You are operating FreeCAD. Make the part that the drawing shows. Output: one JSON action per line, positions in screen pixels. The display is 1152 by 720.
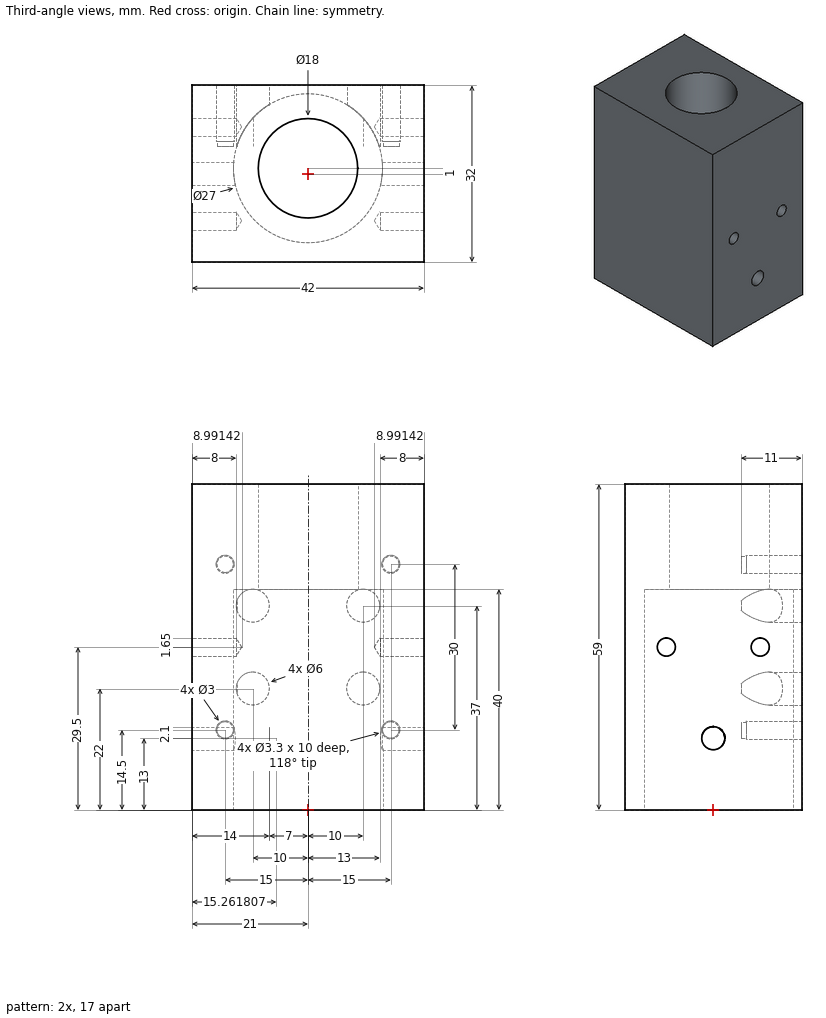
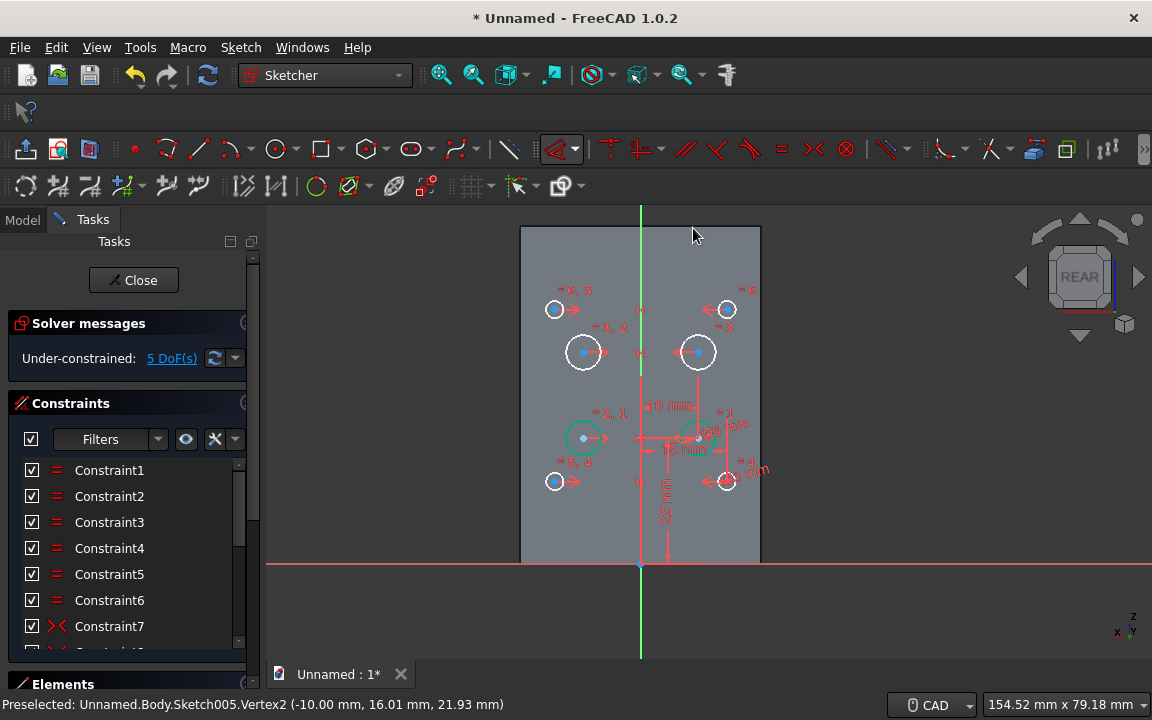
{"action": "left_click", "coordinate": [555, 310]}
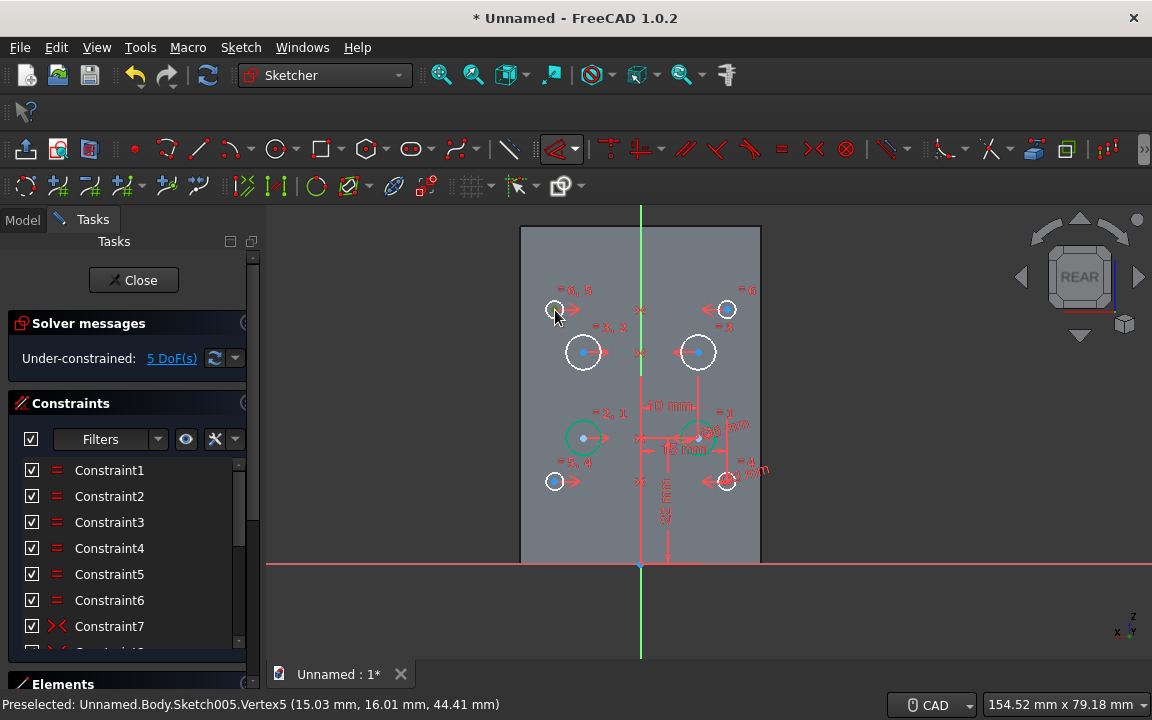
{"action": "key", "text": "l"}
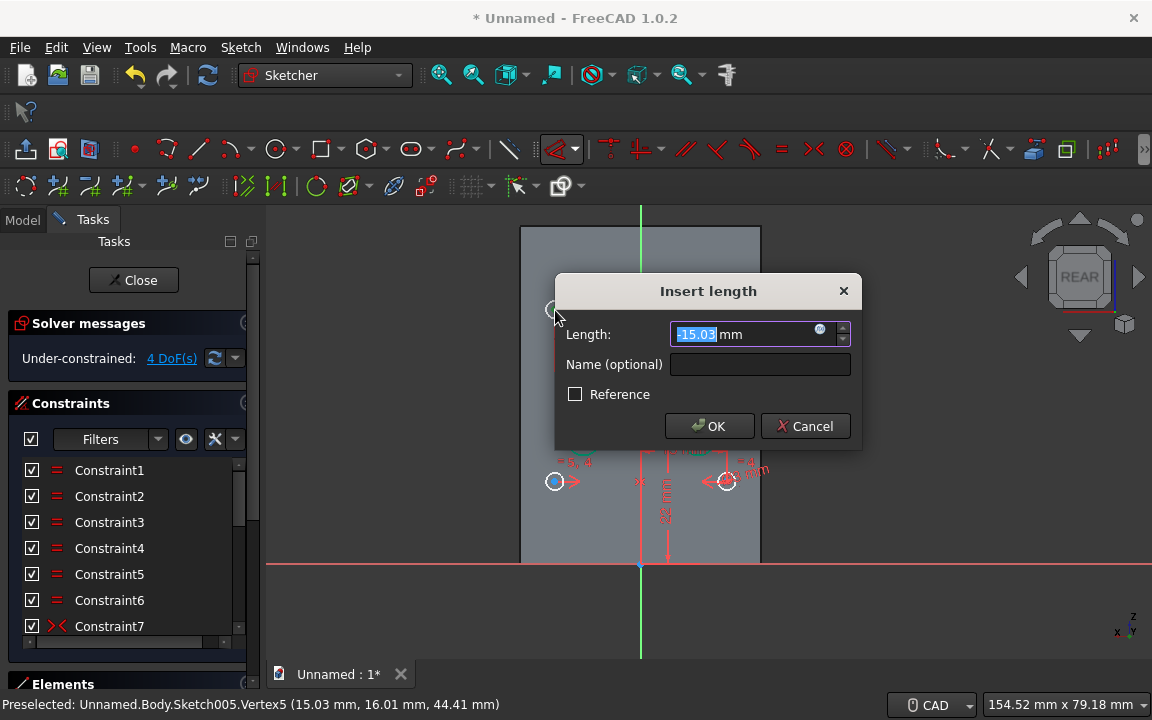
{"action": "type", "text": "-15"}
{"action": "key", "text": "Return"}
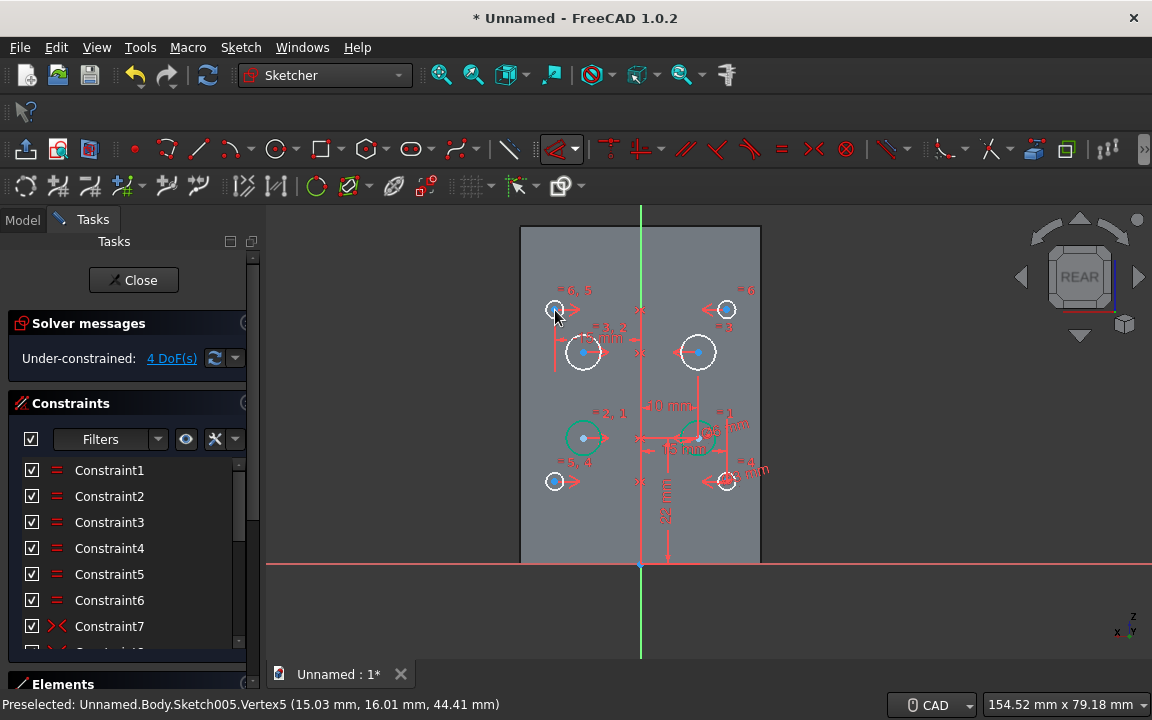
{"action": "left_click", "coordinate": [583, 352]}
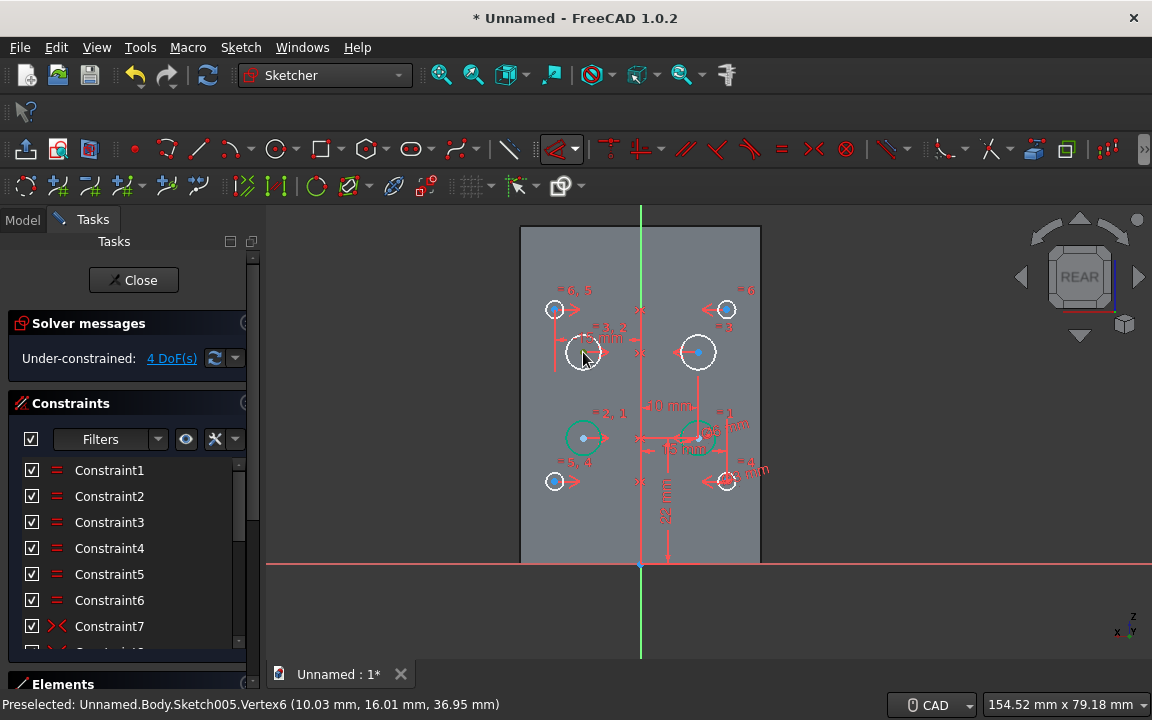
{"action": "key", "text": "l"}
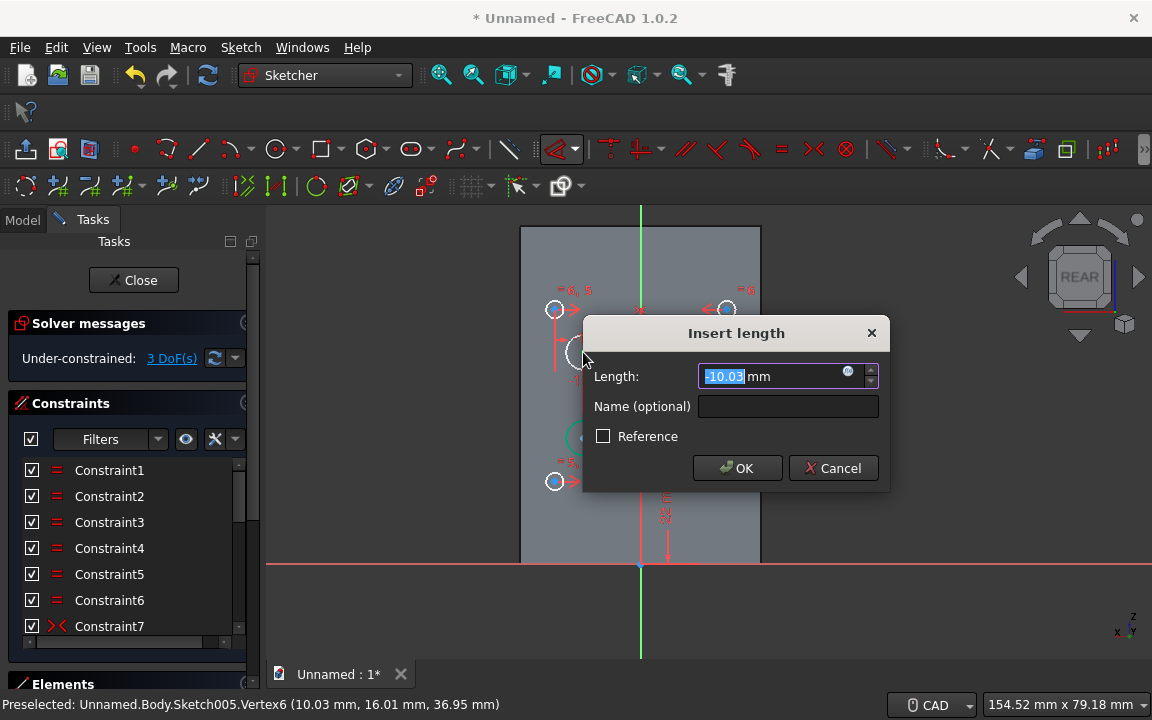
{"action": "type", "text": "-10"}
{"action": "key", "text": "Return"}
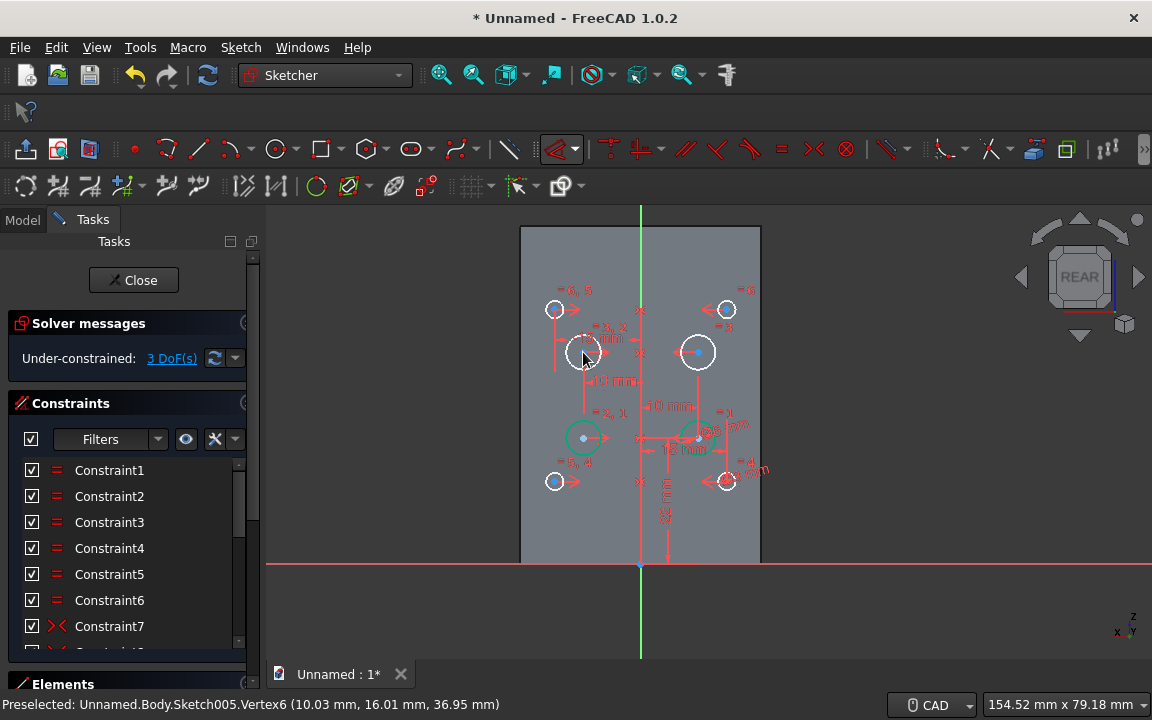
{"action": "left_click", "coordinate": [584, 352]}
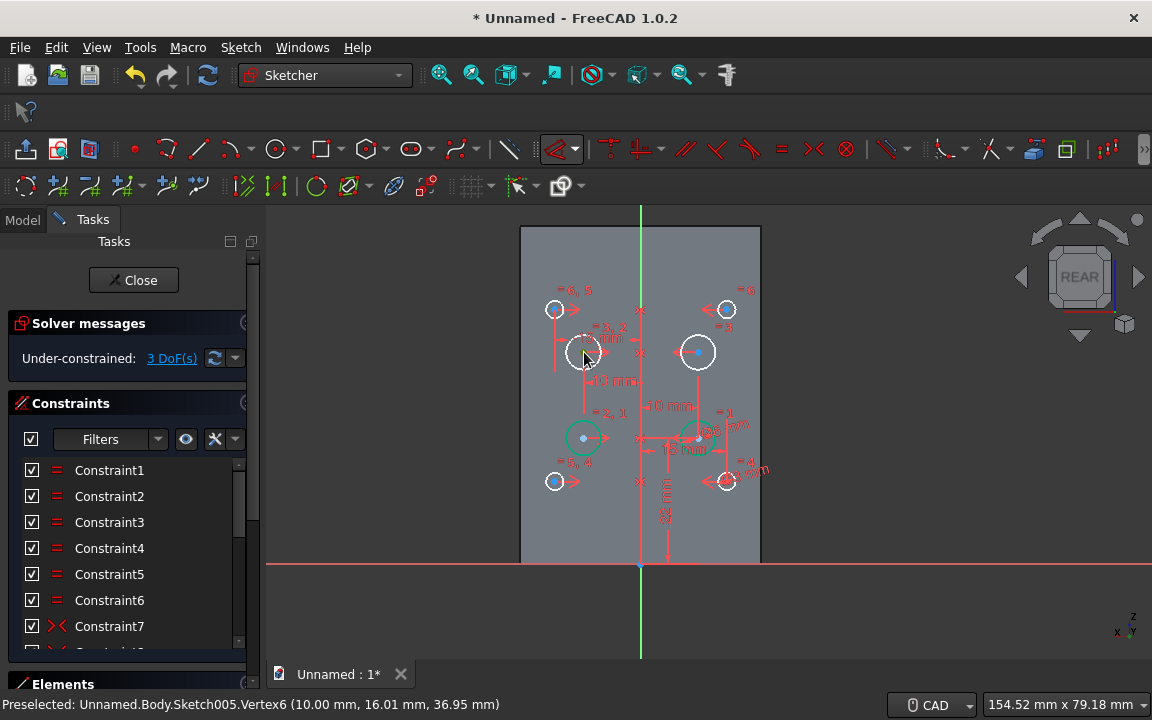
{"action": "key", "text": "i"}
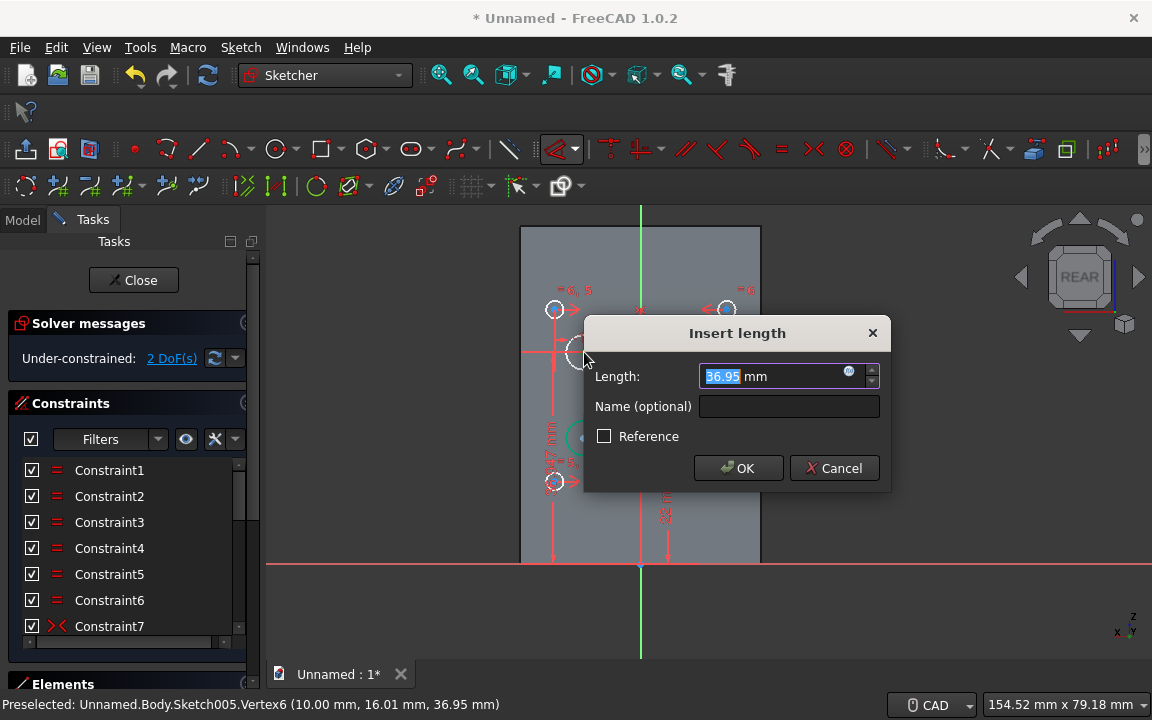
{"action": "type", "text": "37"}
{"action": "key", "text": "Return"}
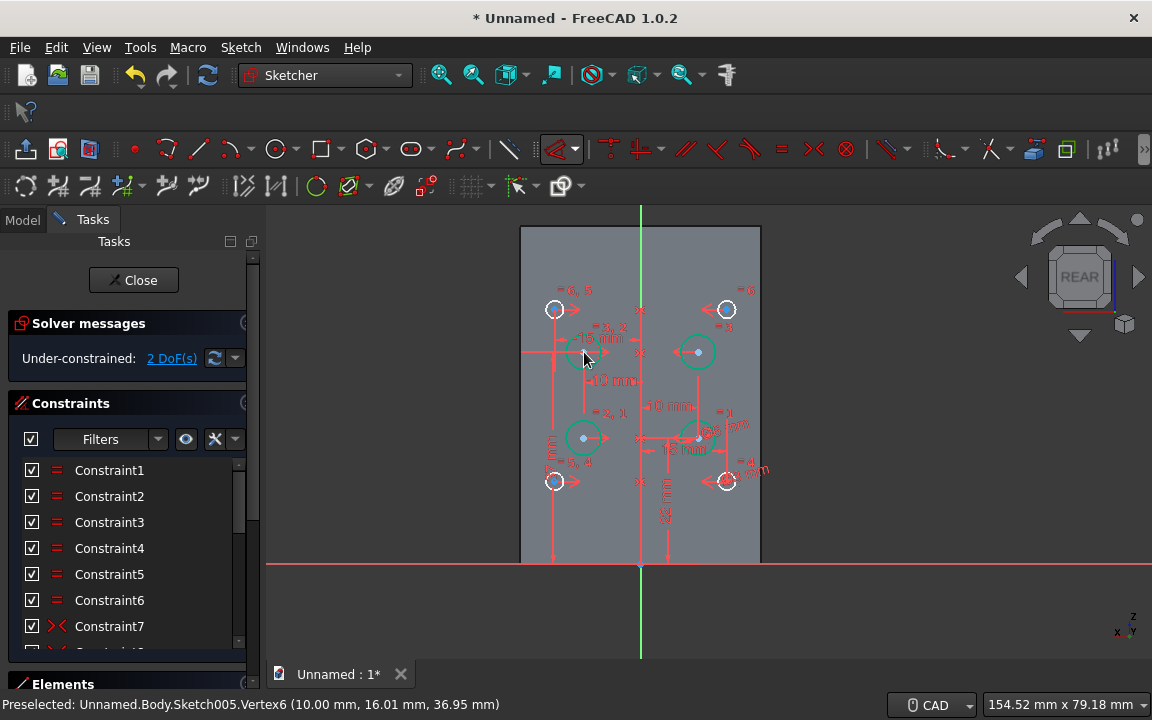
{"action": "left_click", "coordinate": [555, 482]}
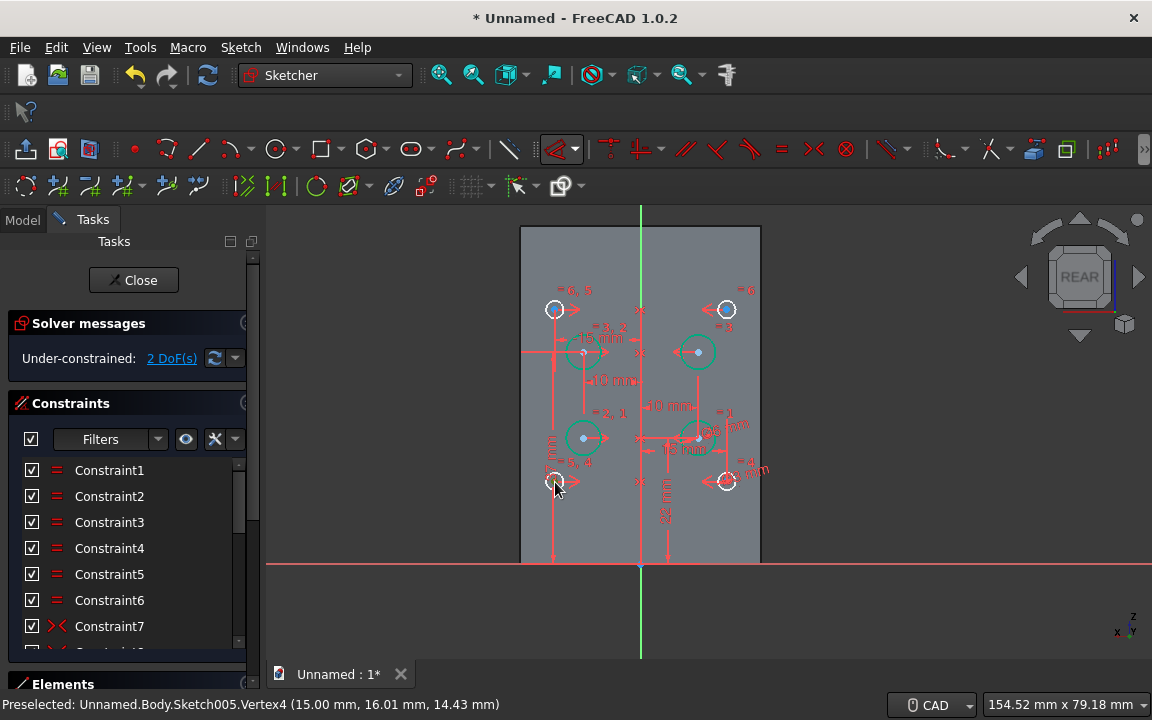
{"action": "left_click", "coordinate": [555, 310]}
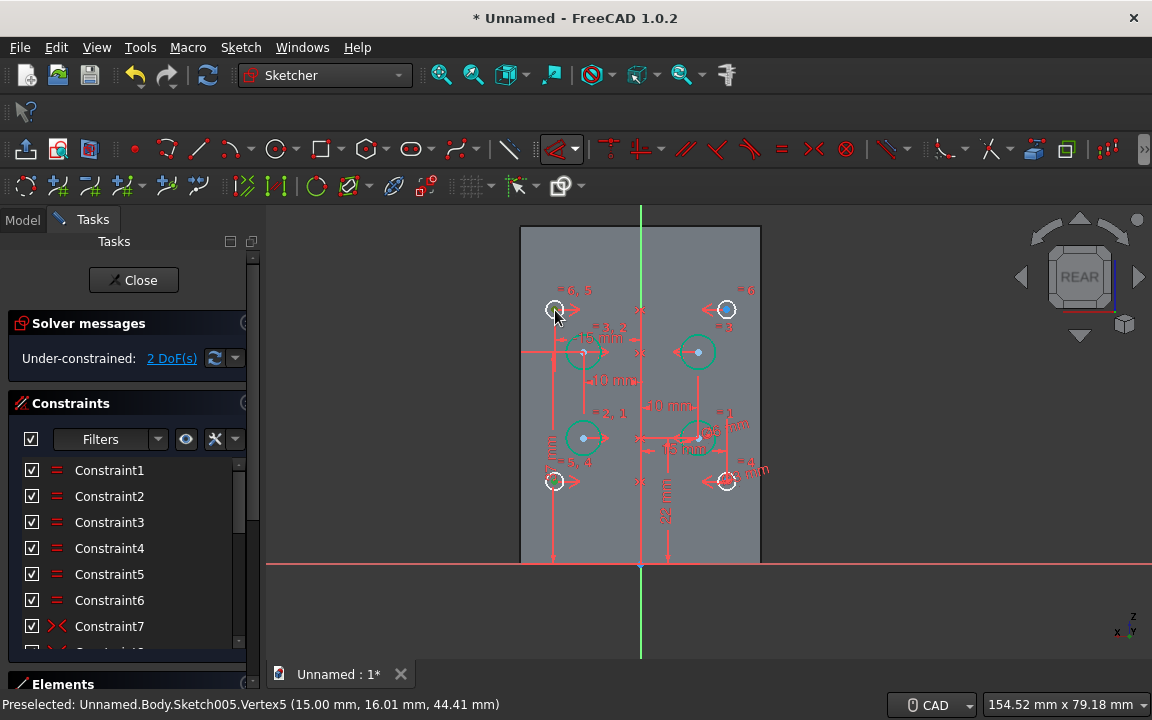
{"action": "key", "text": "i"}